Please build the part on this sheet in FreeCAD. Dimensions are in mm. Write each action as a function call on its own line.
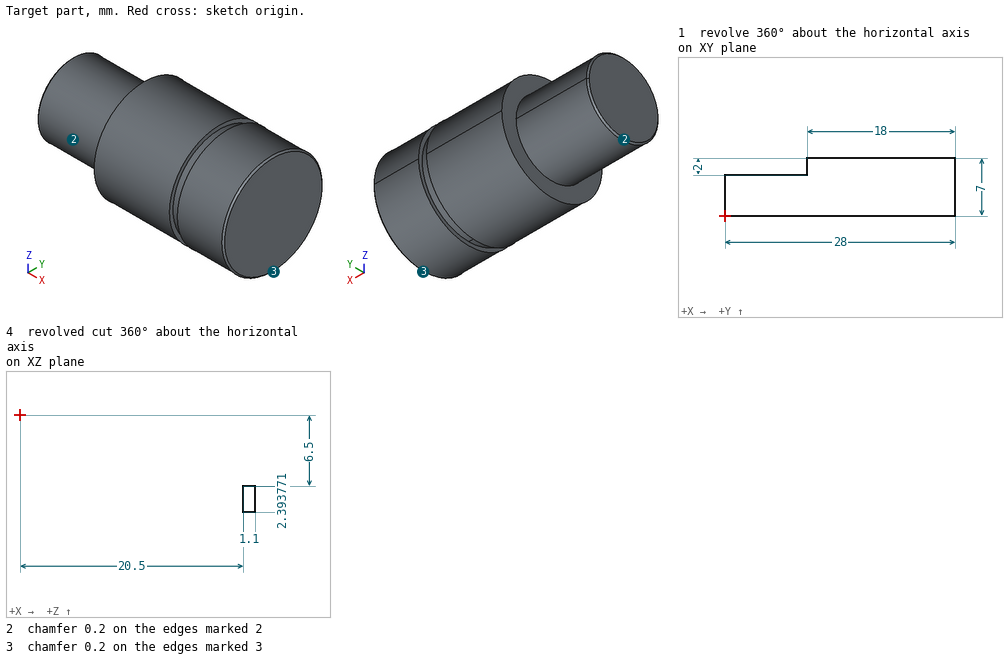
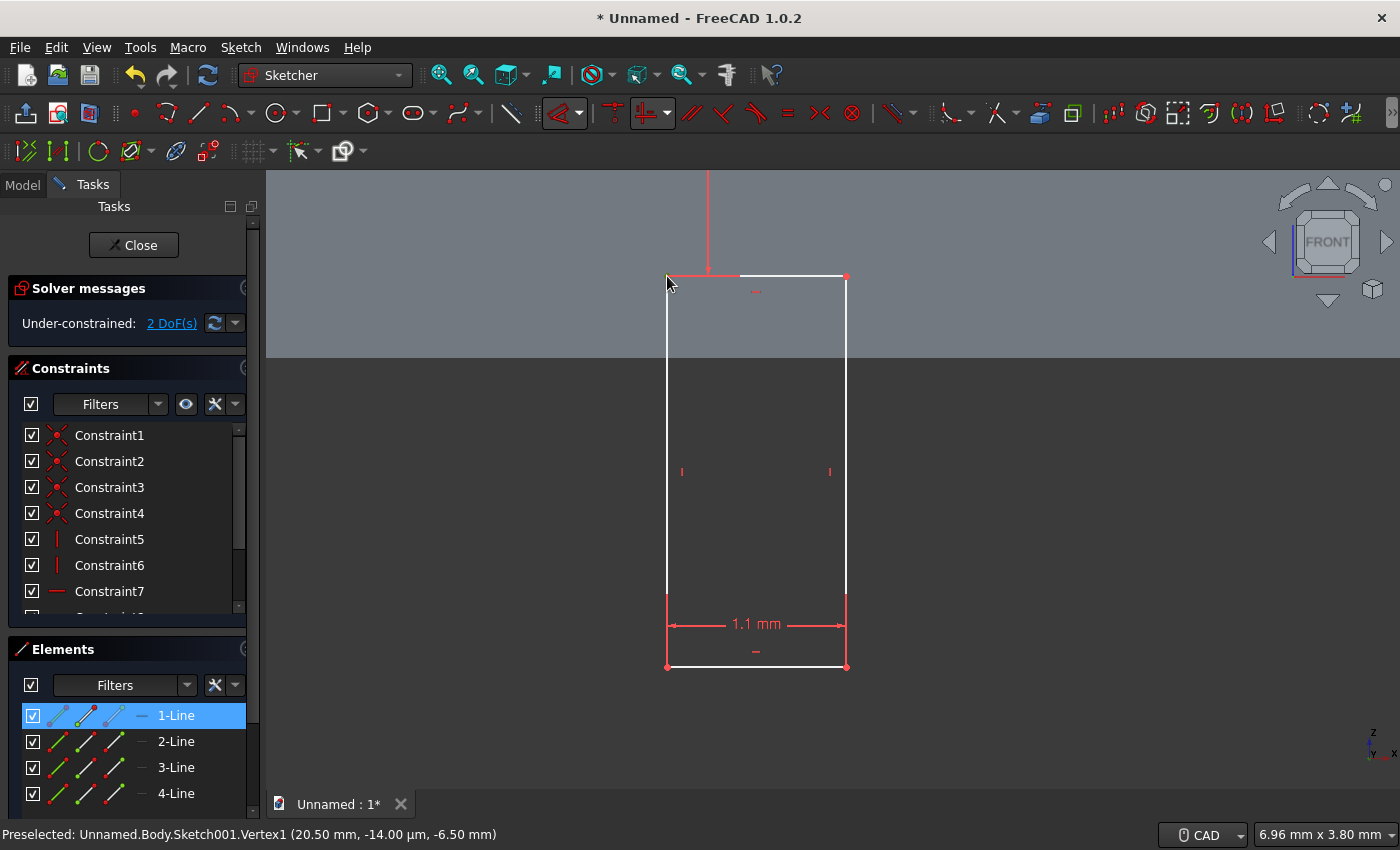
click(582, 114)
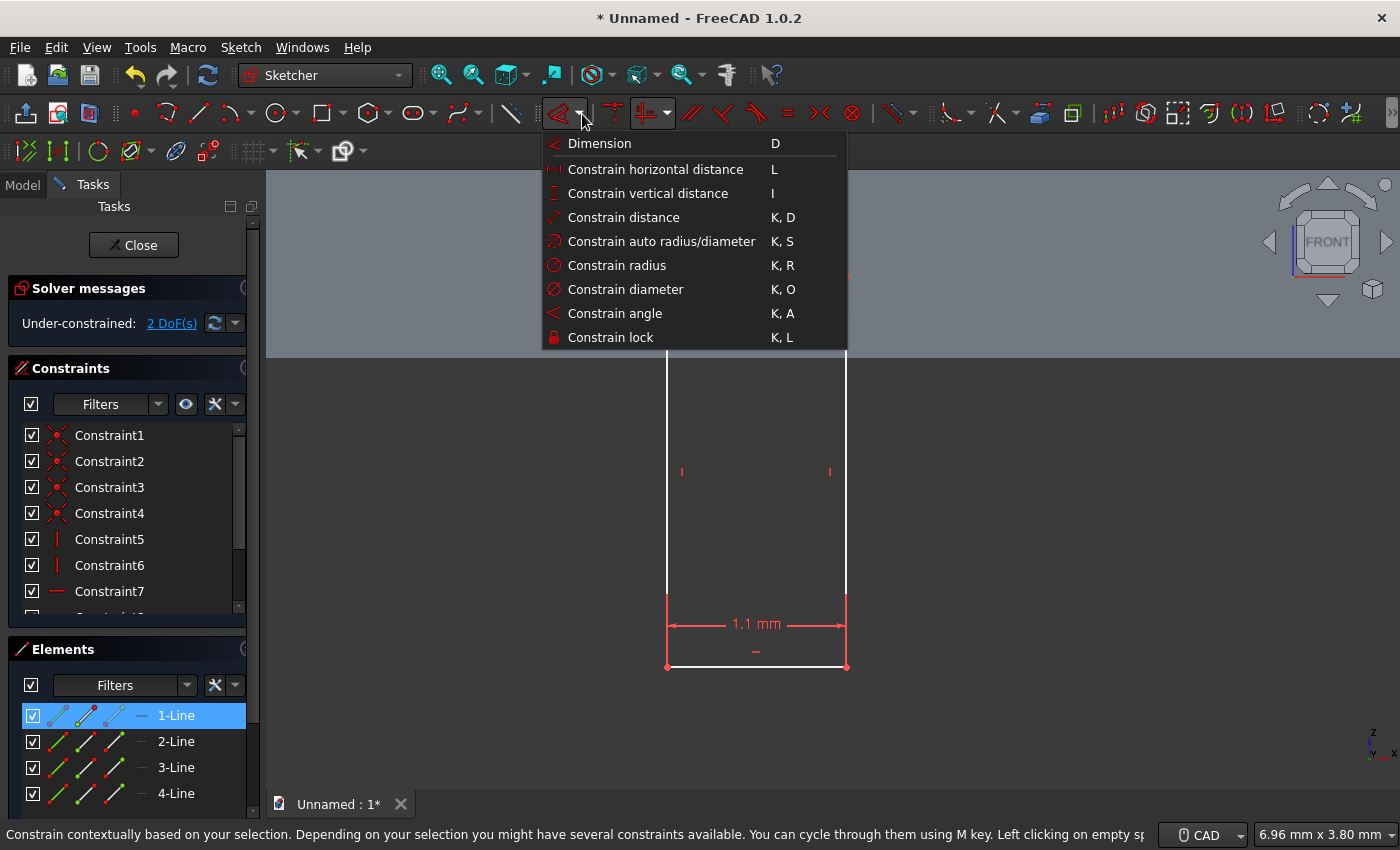
click(695, 169)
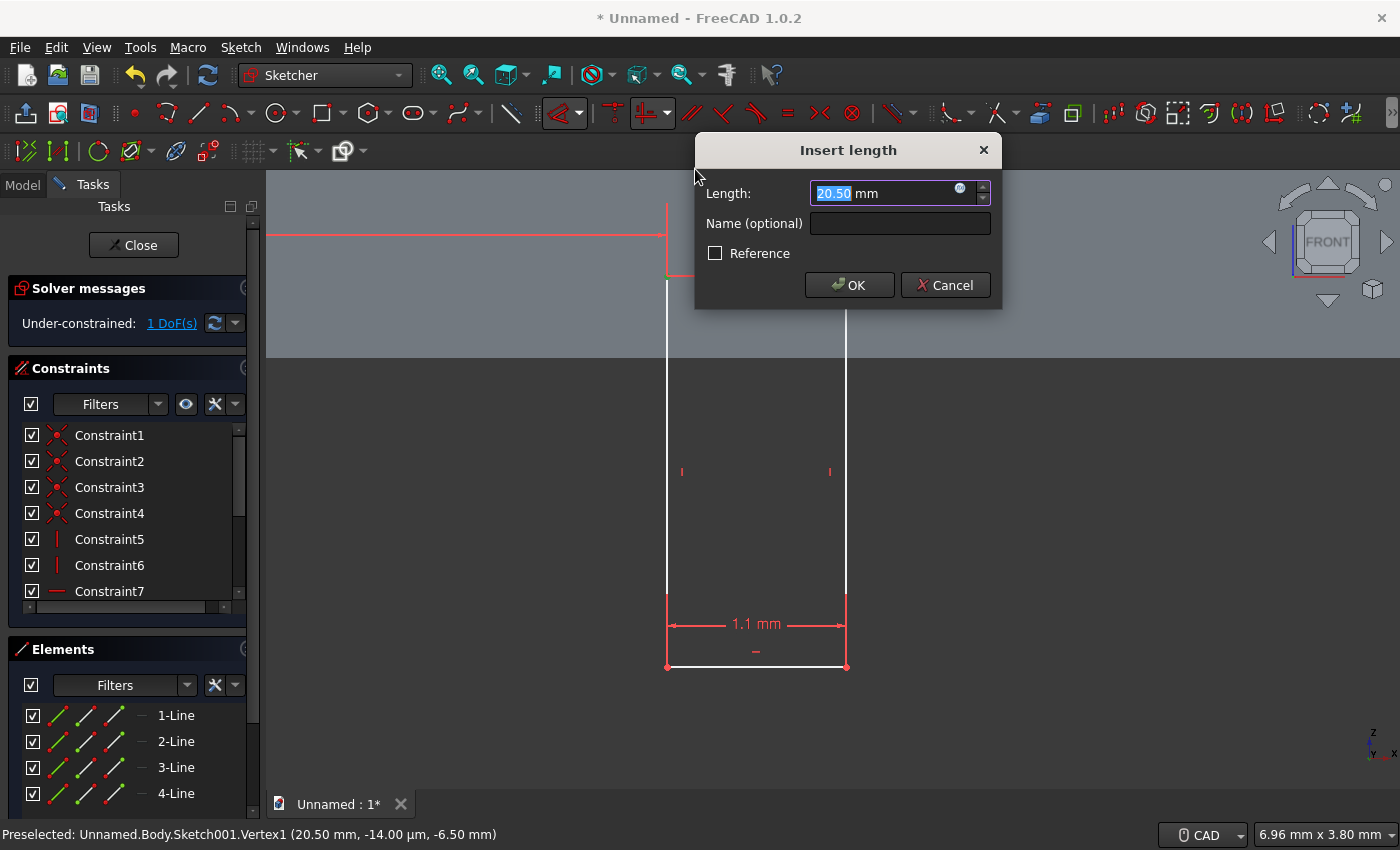
text(20.5)
key(Return)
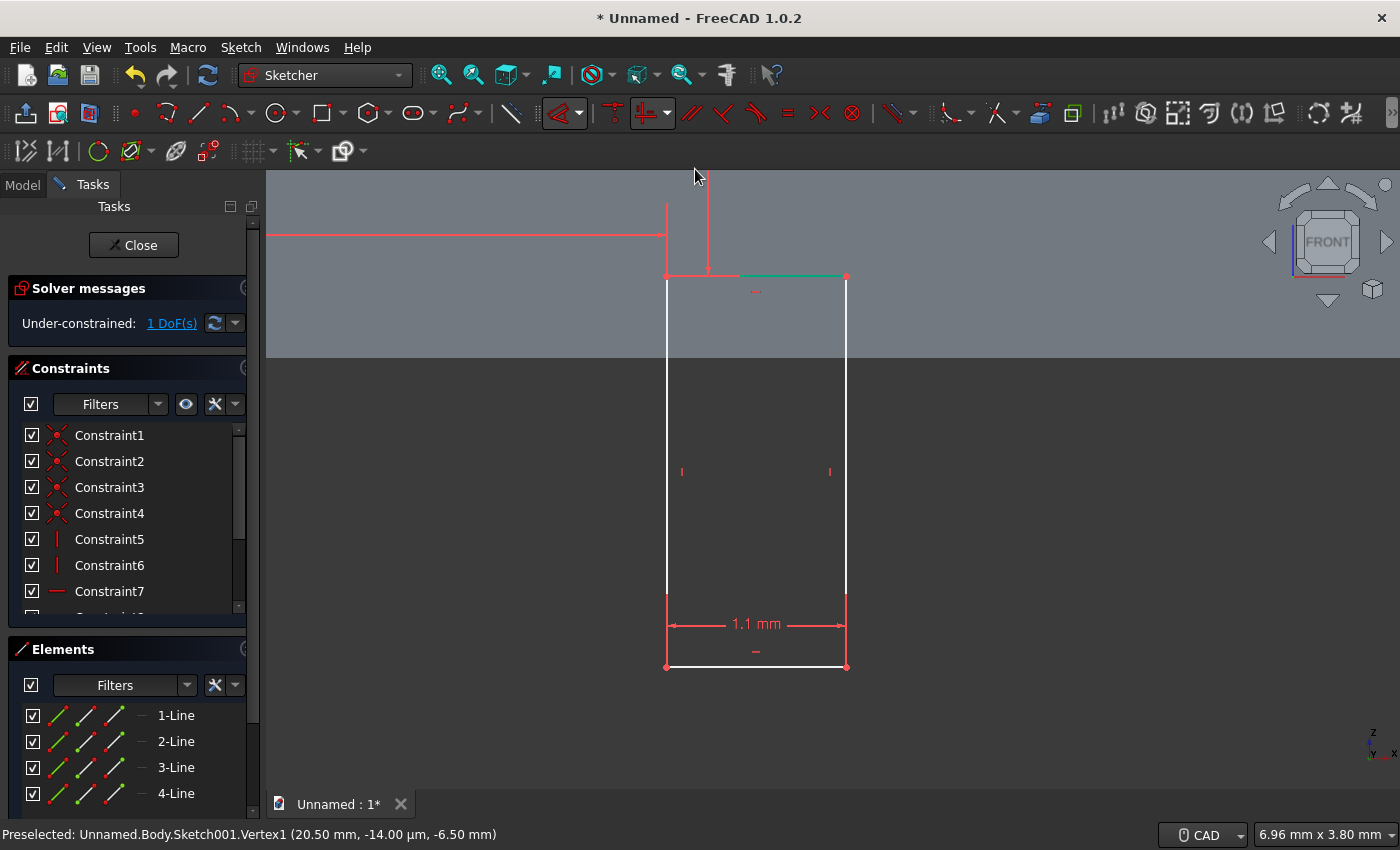
click(667, 394)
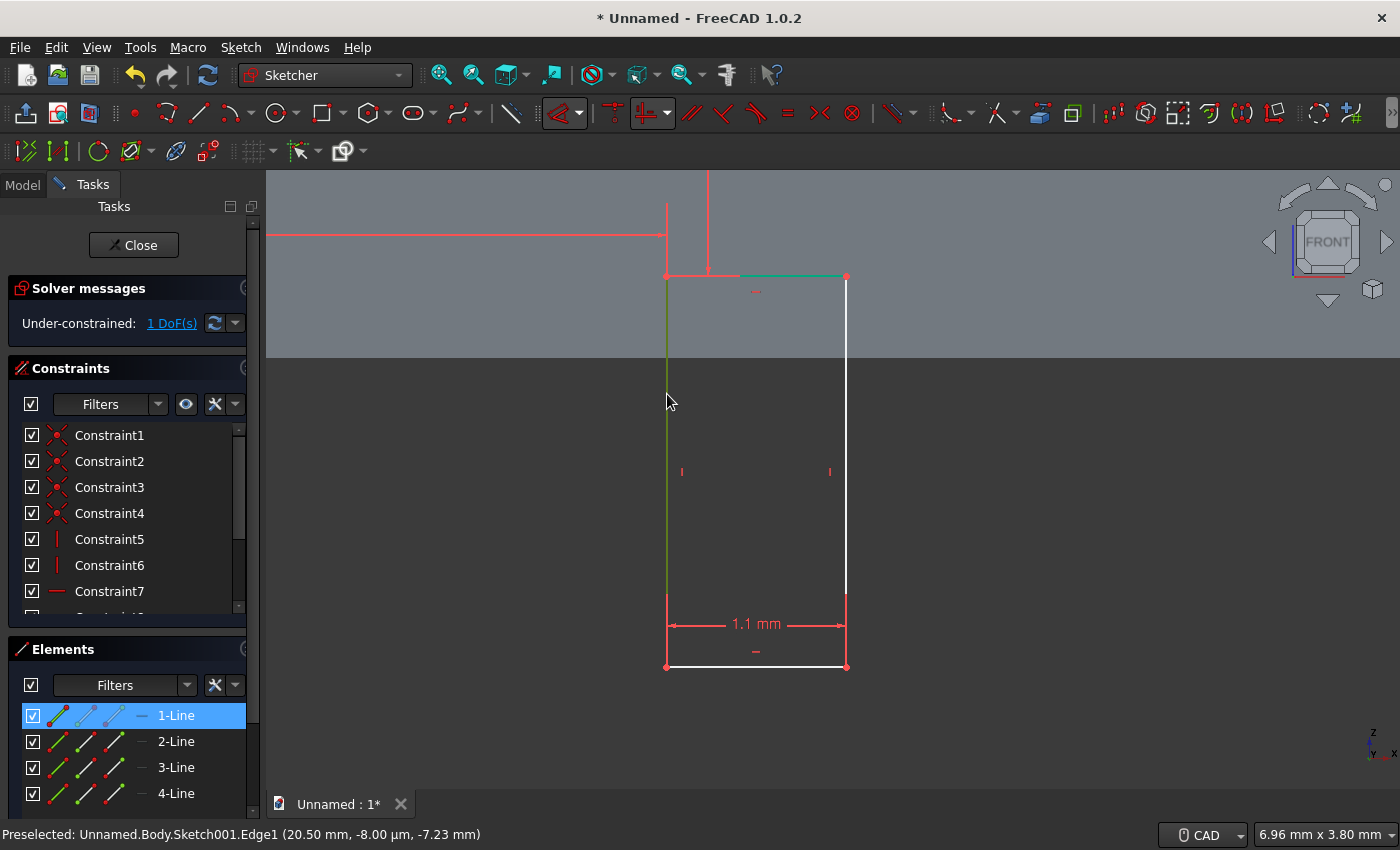
key(i)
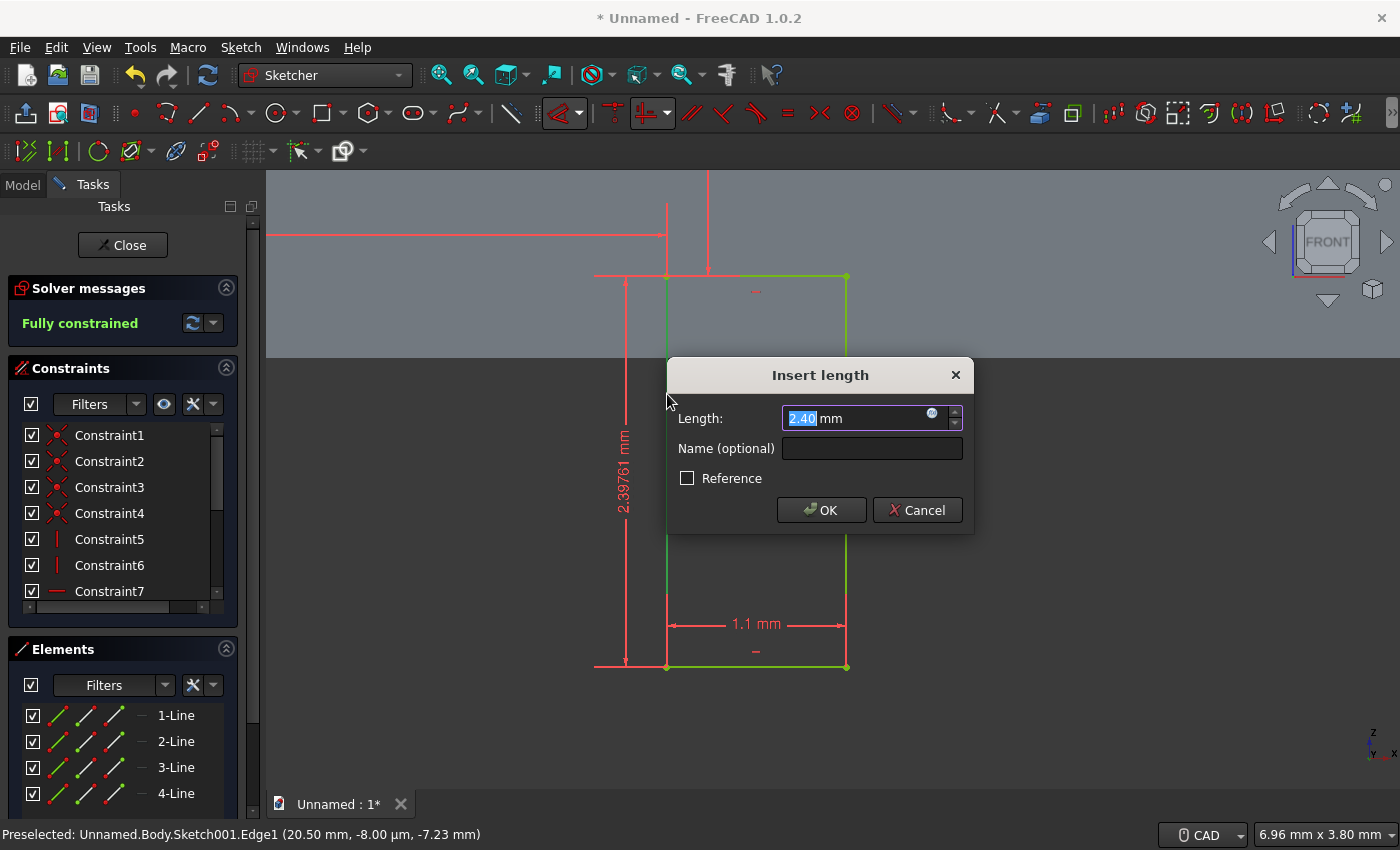
text(2.393771)
key(Return)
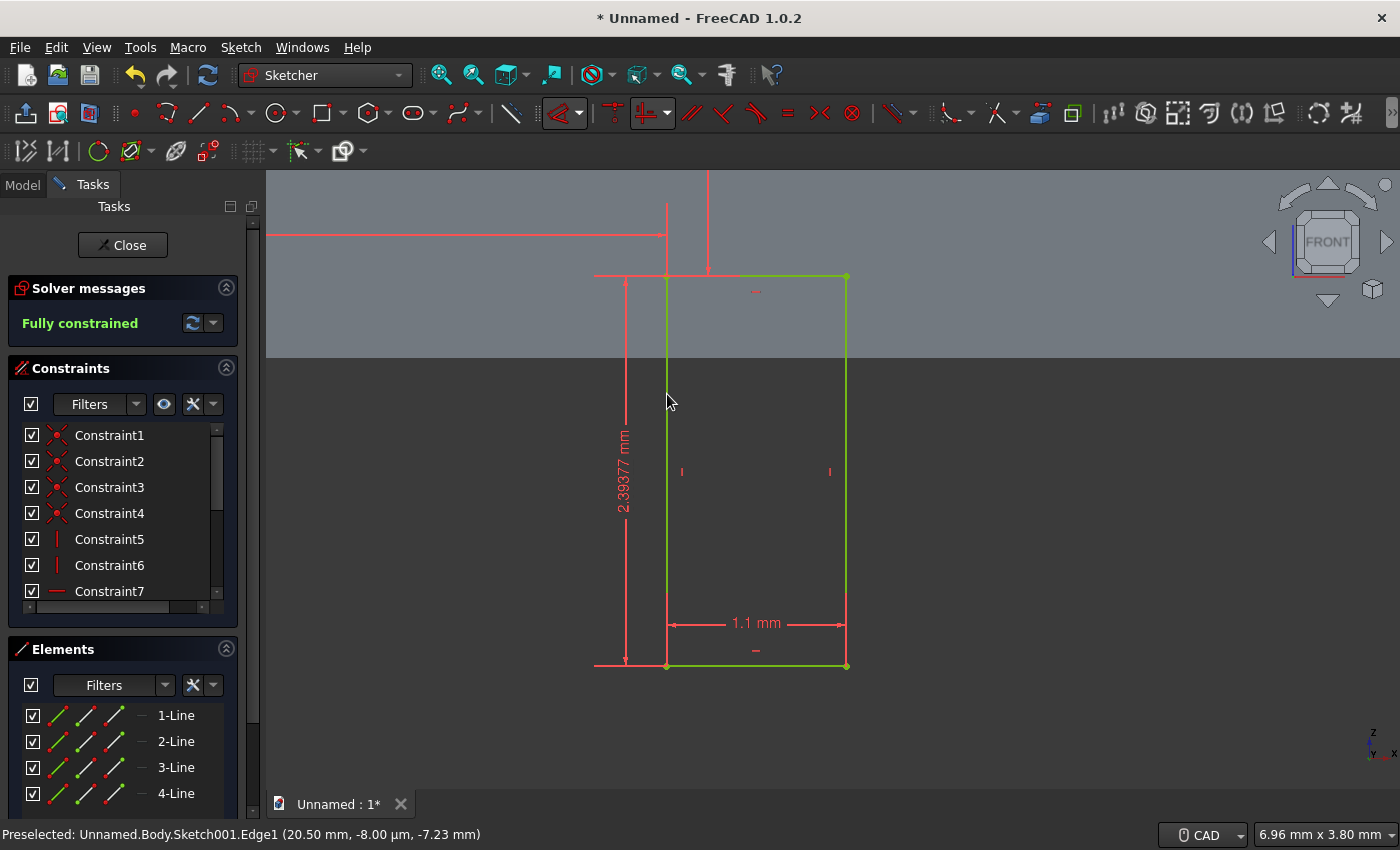
click(123, 245)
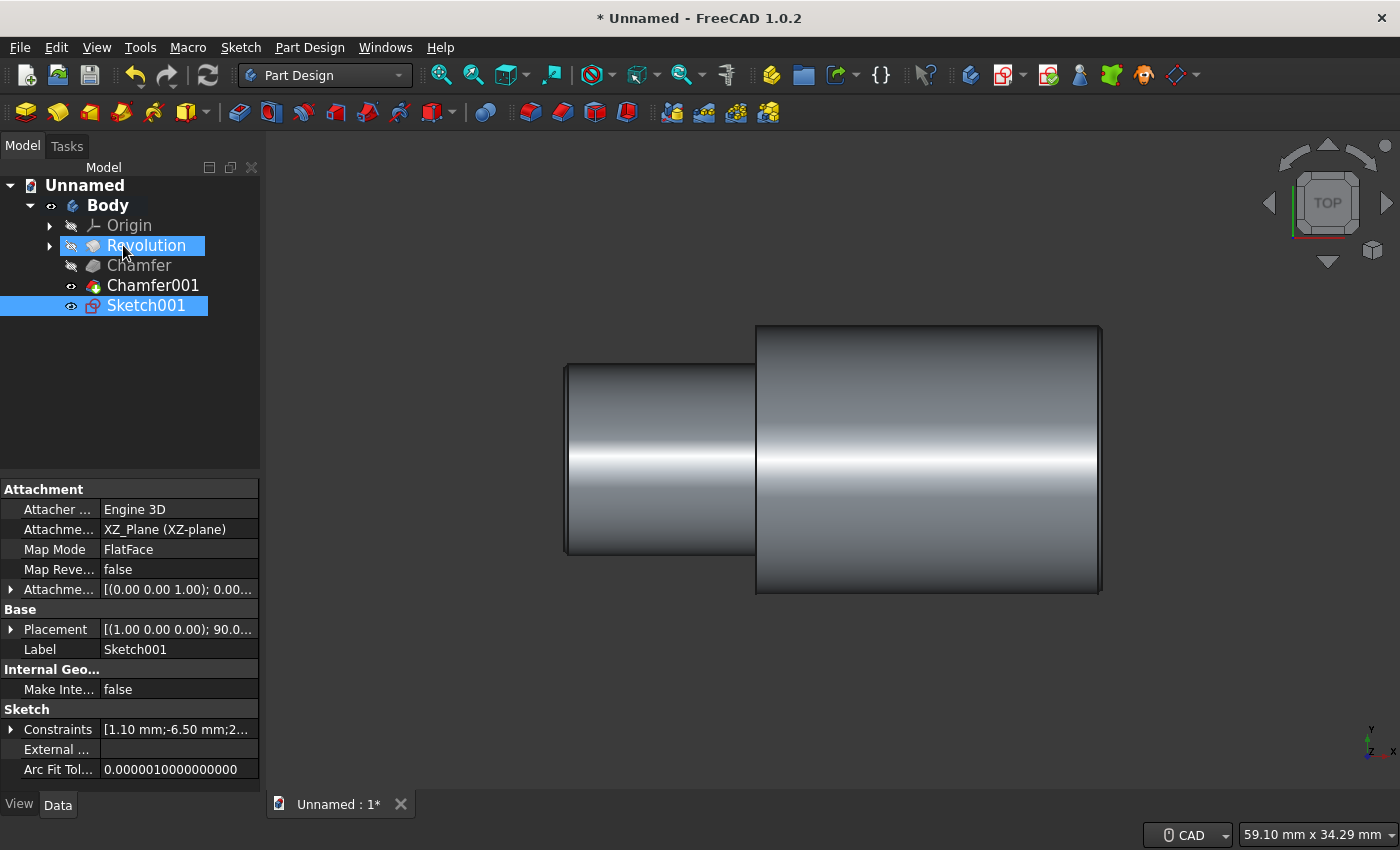
click(304, 112)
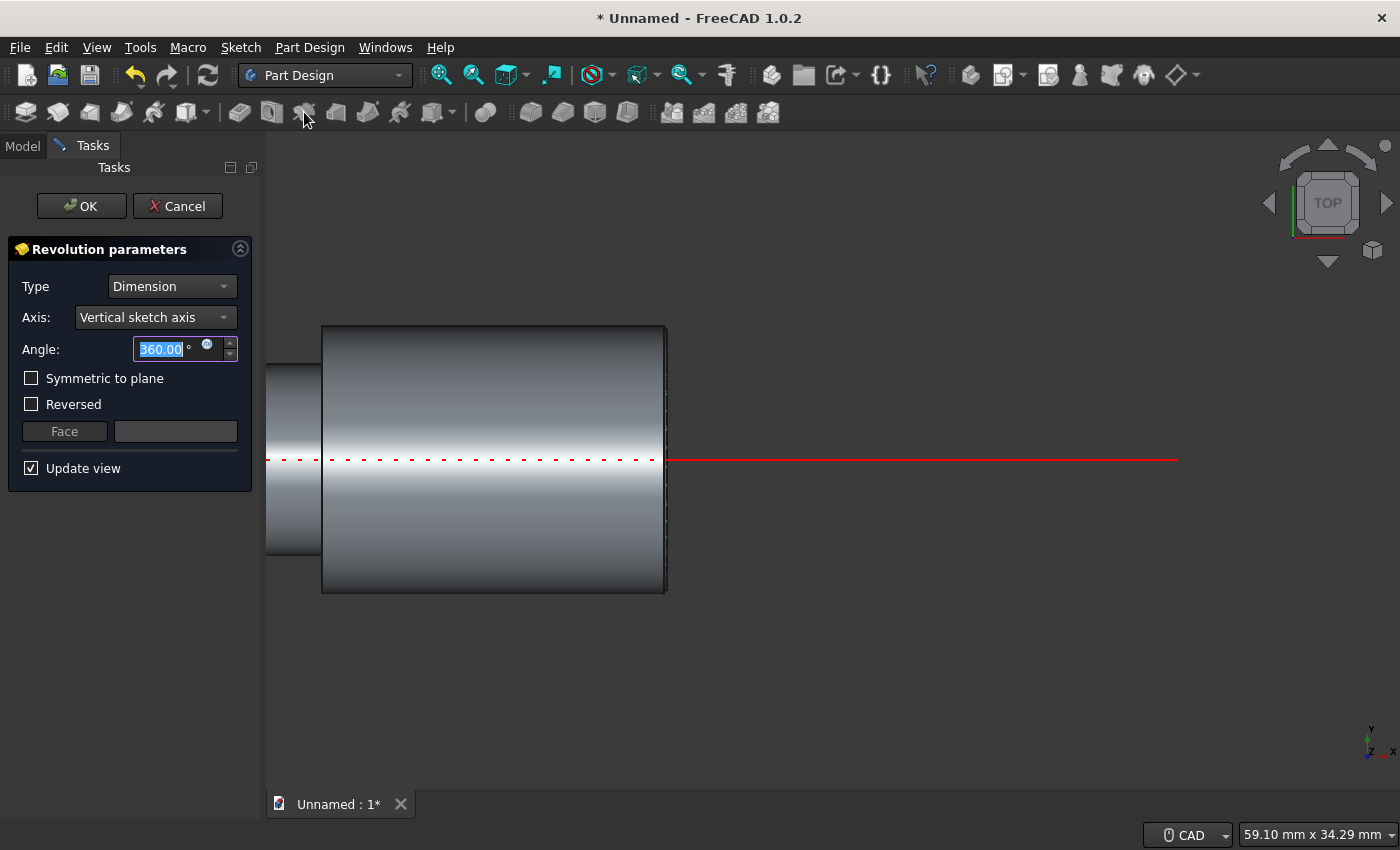
click(156, 318)